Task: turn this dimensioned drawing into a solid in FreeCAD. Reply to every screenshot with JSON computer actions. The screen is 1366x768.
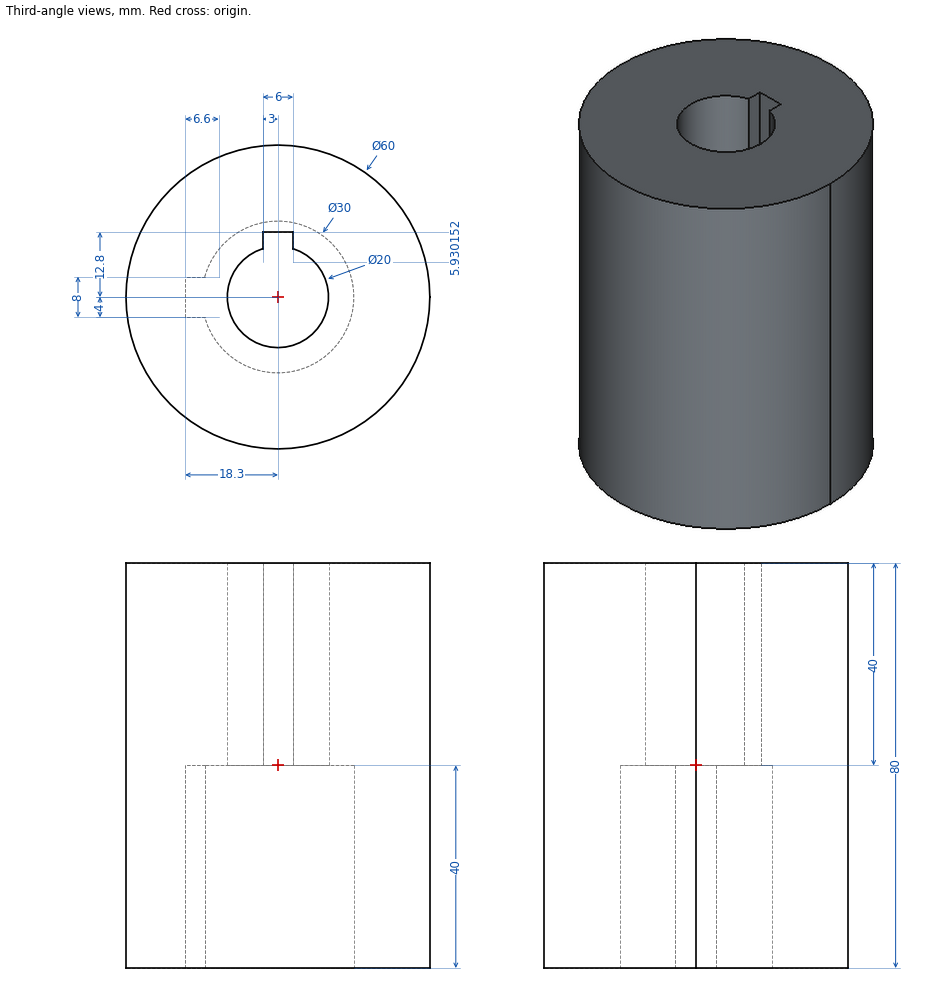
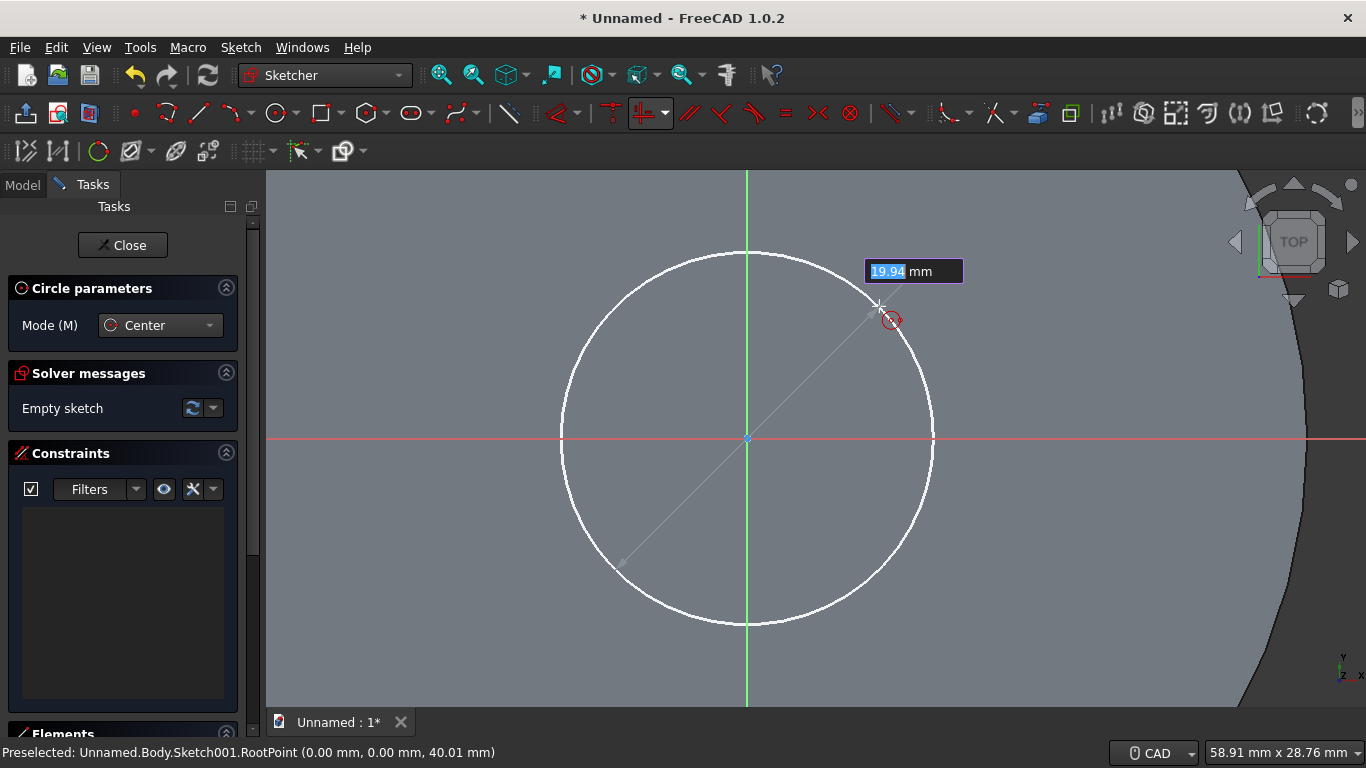
{"action": "type", "text": "20"}
{"action": "key", "text": "Return"}
{"action": "key", "text": "Escape"}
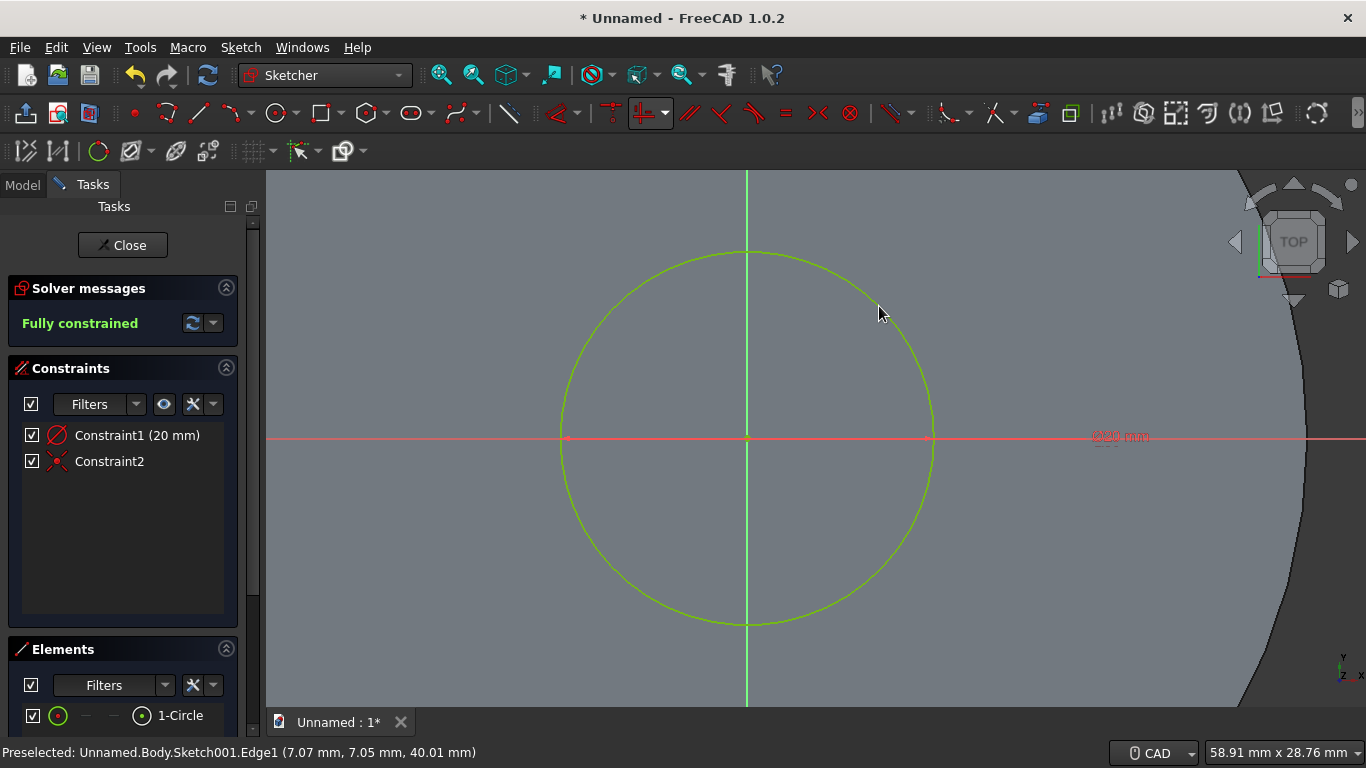
{"action": "left_click", "coordinate": [123, 245]}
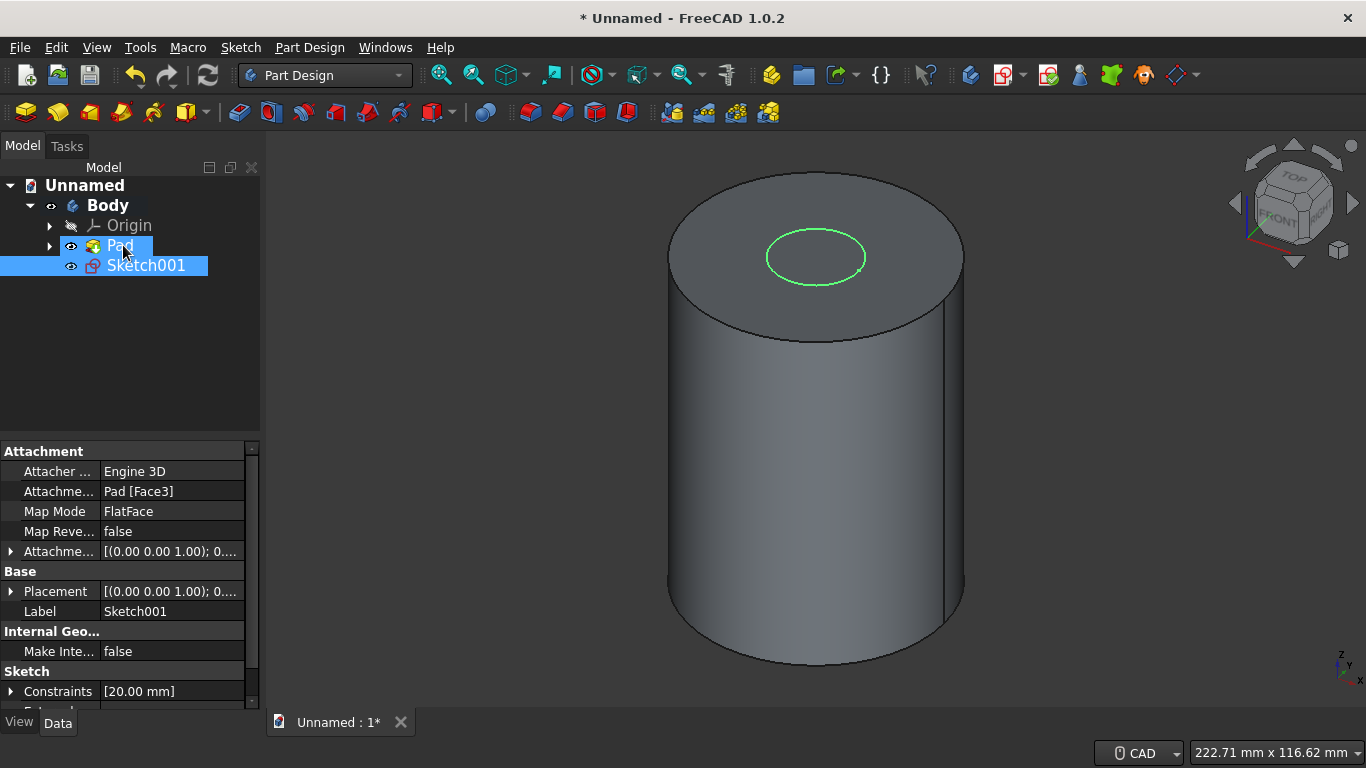
{"action": "left_click", "coordinate": [240, 112]}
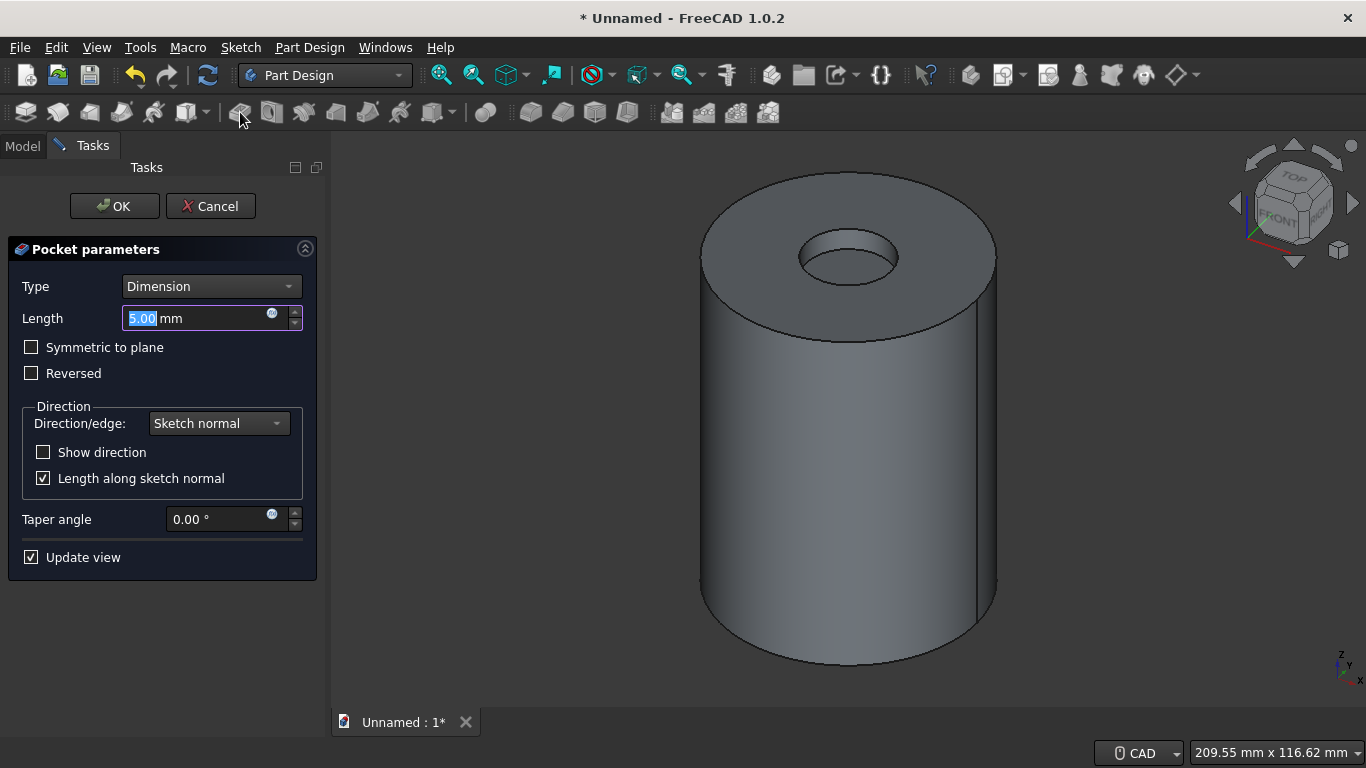
{"action": "left_click", "coordinate": [212, 286]}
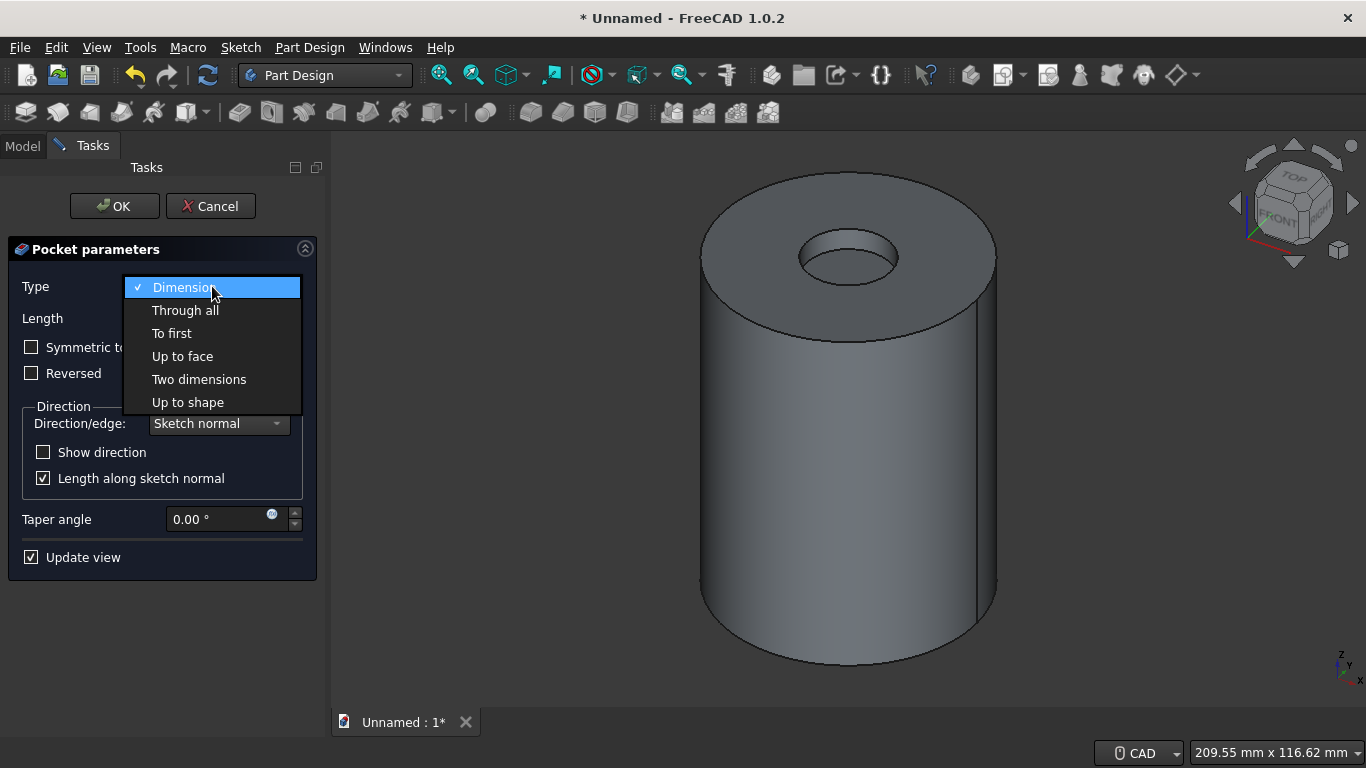
{"action": "left_click", "coordinate": [212, 310]}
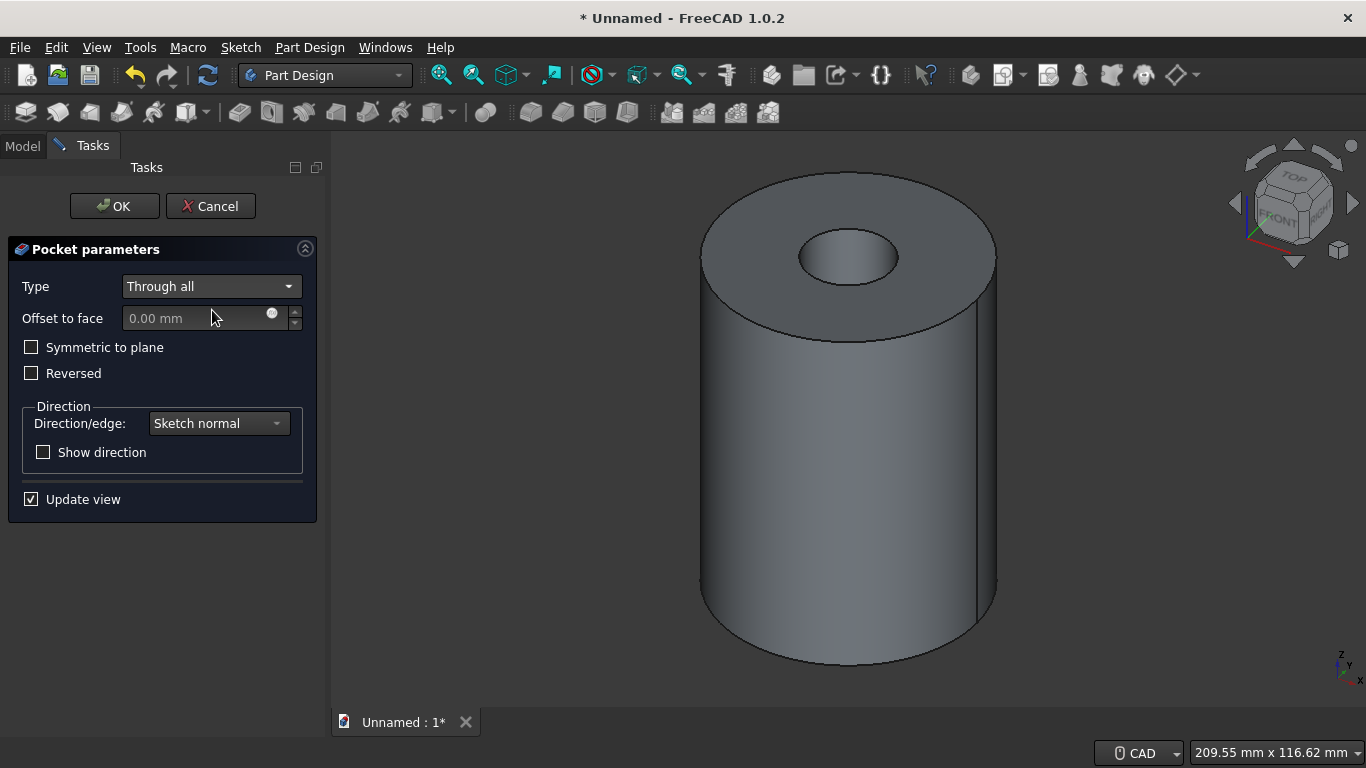
{"action": "left_click", "coordinate": [115, 206]}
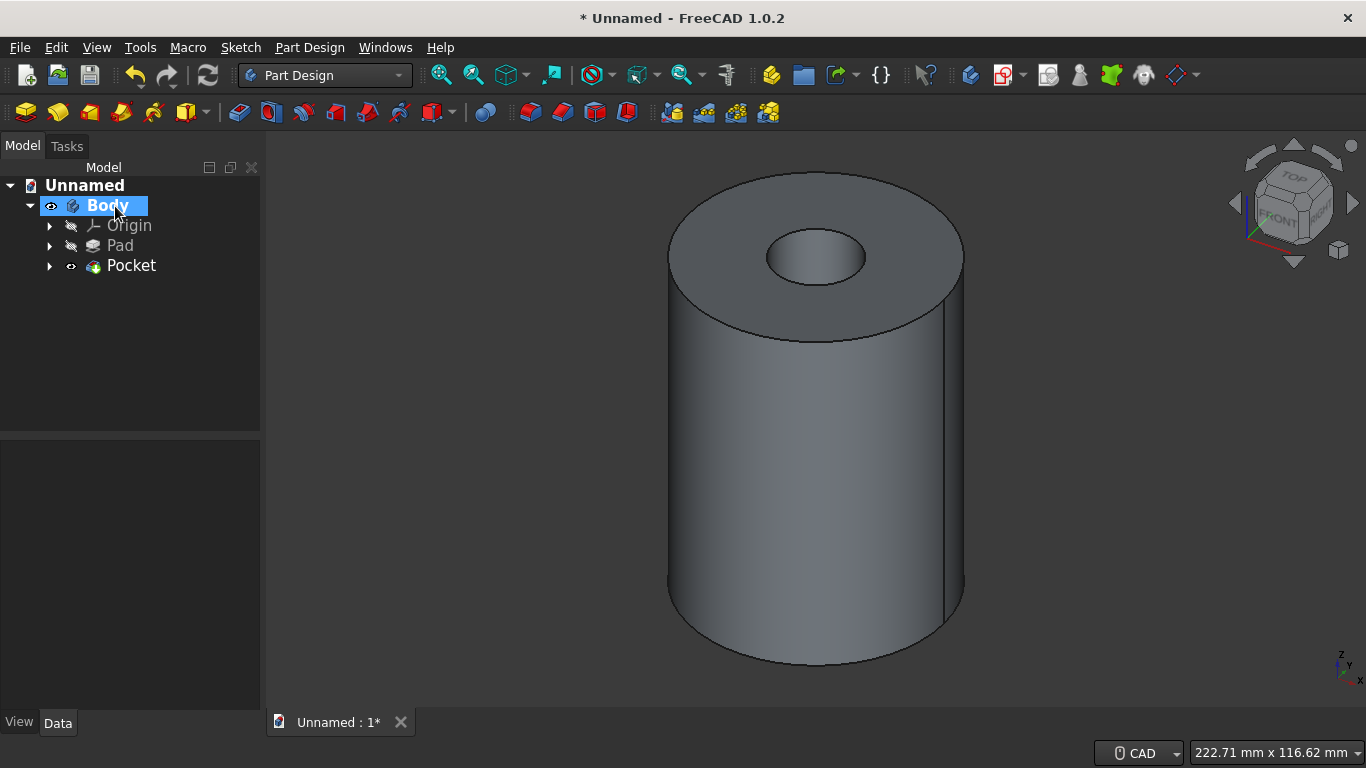
{"action": "key", "text": "5"}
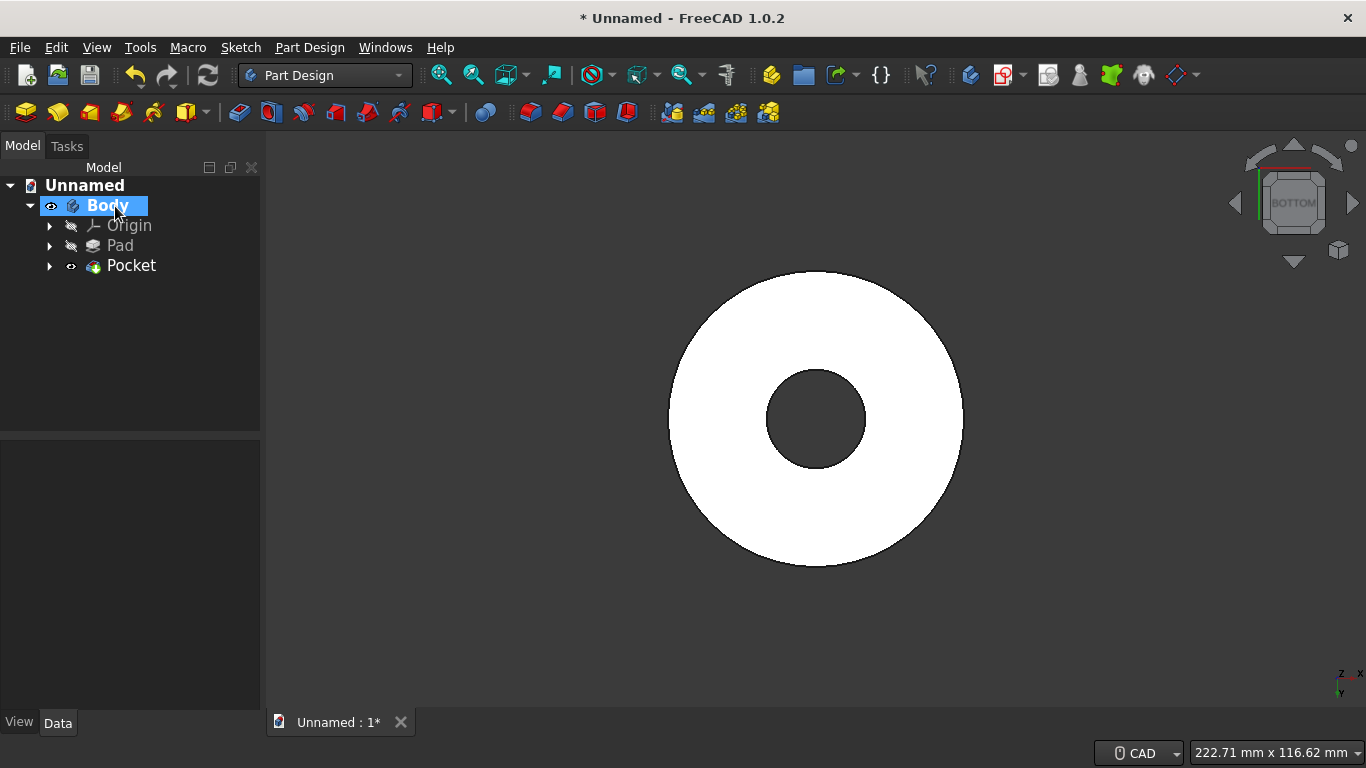
{"action": "left_click", "coordinate": [774, 503]}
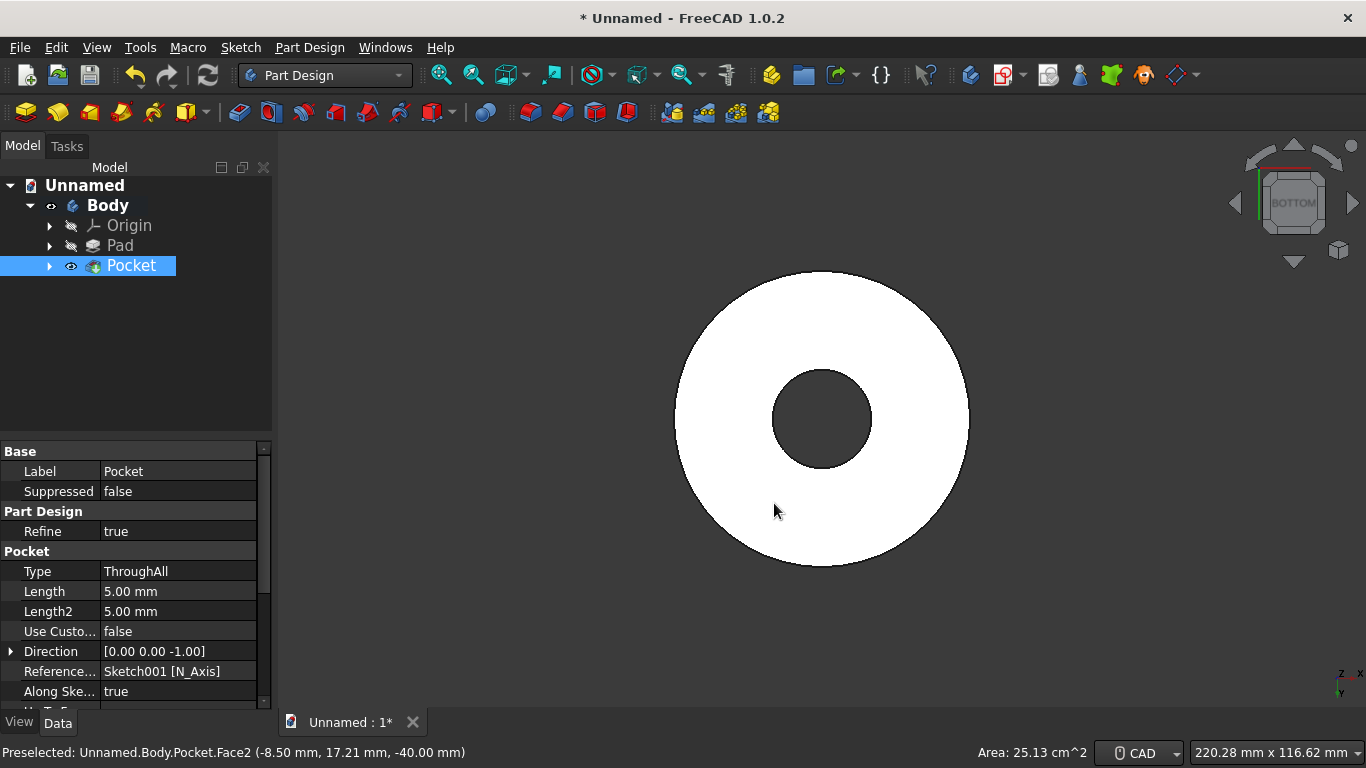
{"action": "left_click", "coordinate": [1004, 76]}